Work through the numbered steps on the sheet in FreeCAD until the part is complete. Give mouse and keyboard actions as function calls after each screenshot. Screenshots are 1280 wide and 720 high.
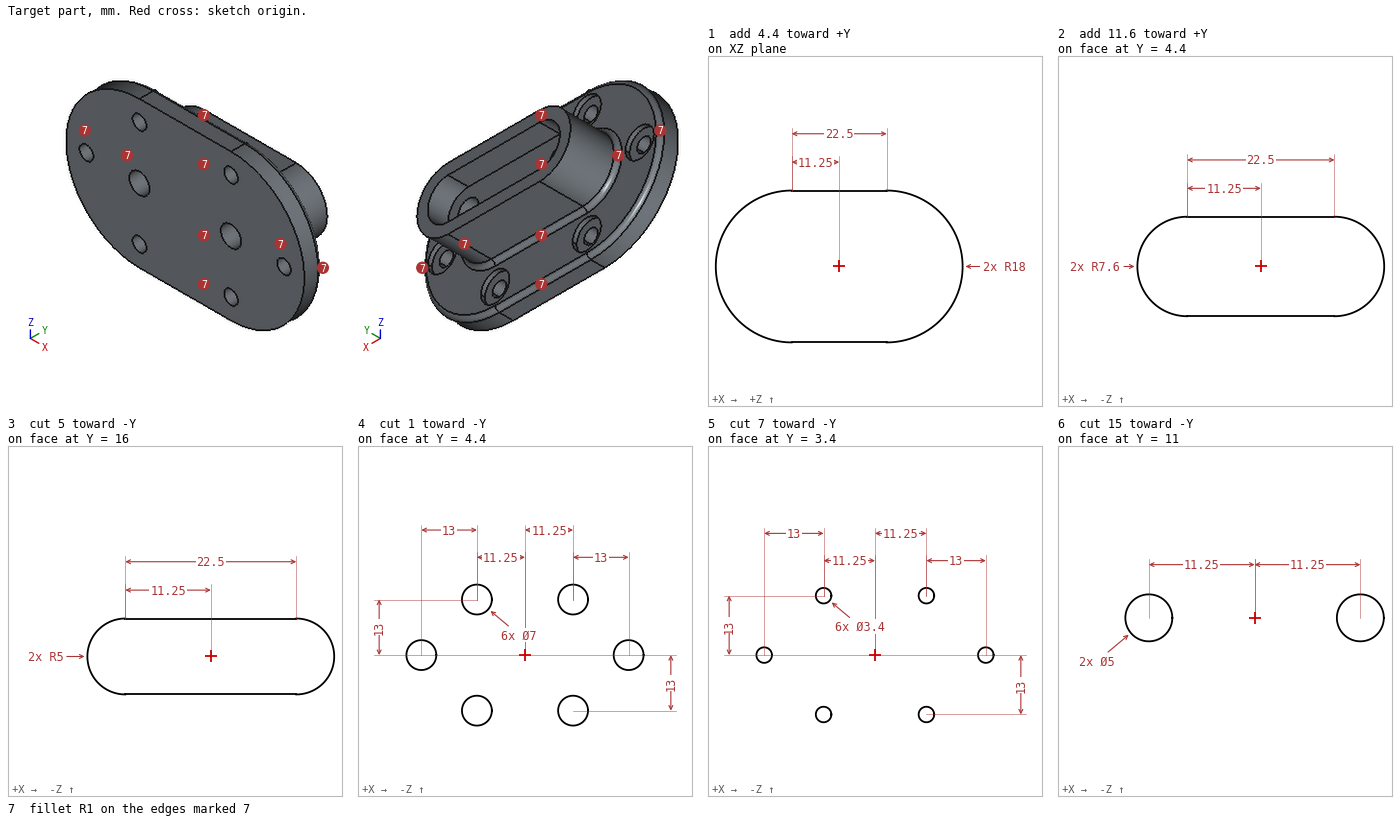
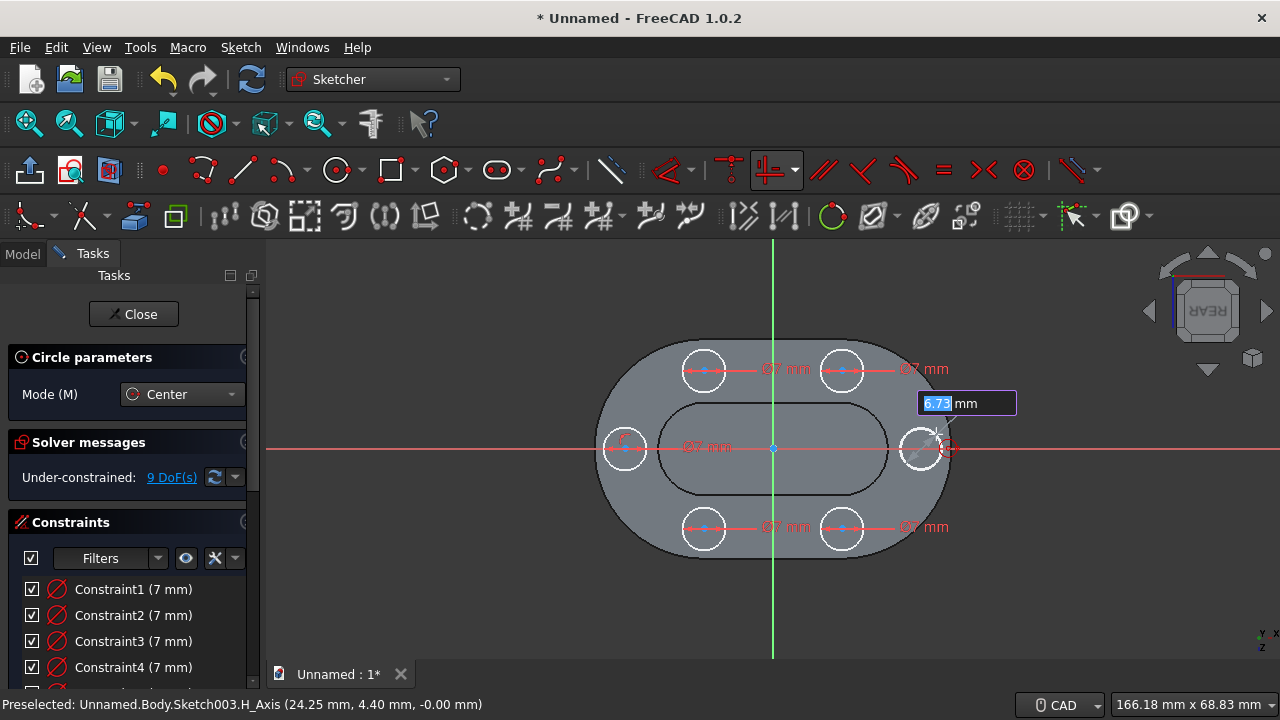
text(7)
key(Return)
key(Escape)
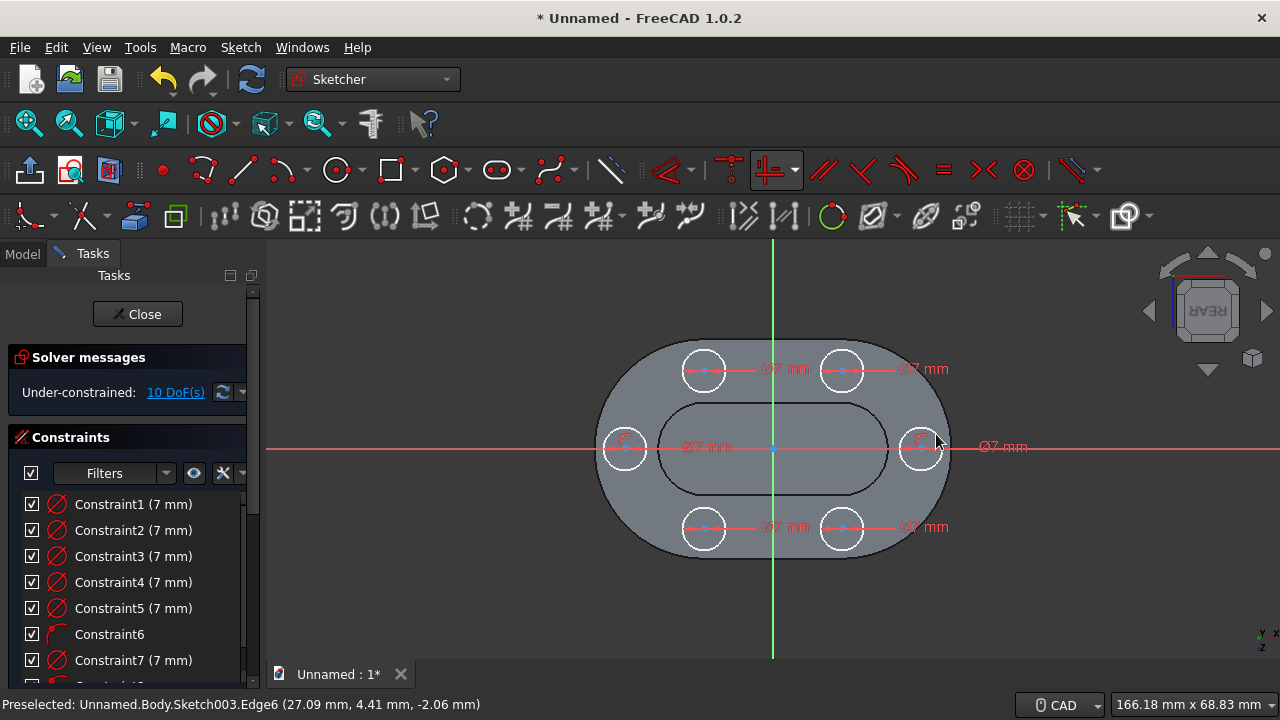
click(704, 371)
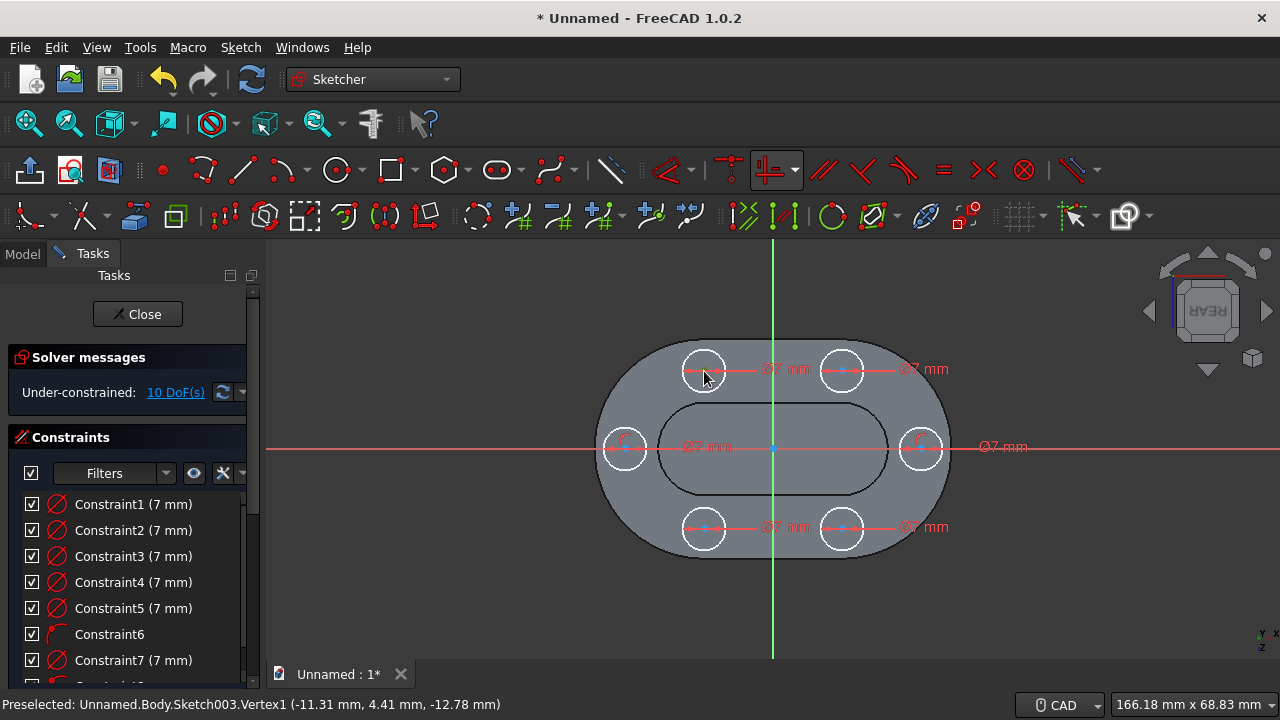
click(842, 371)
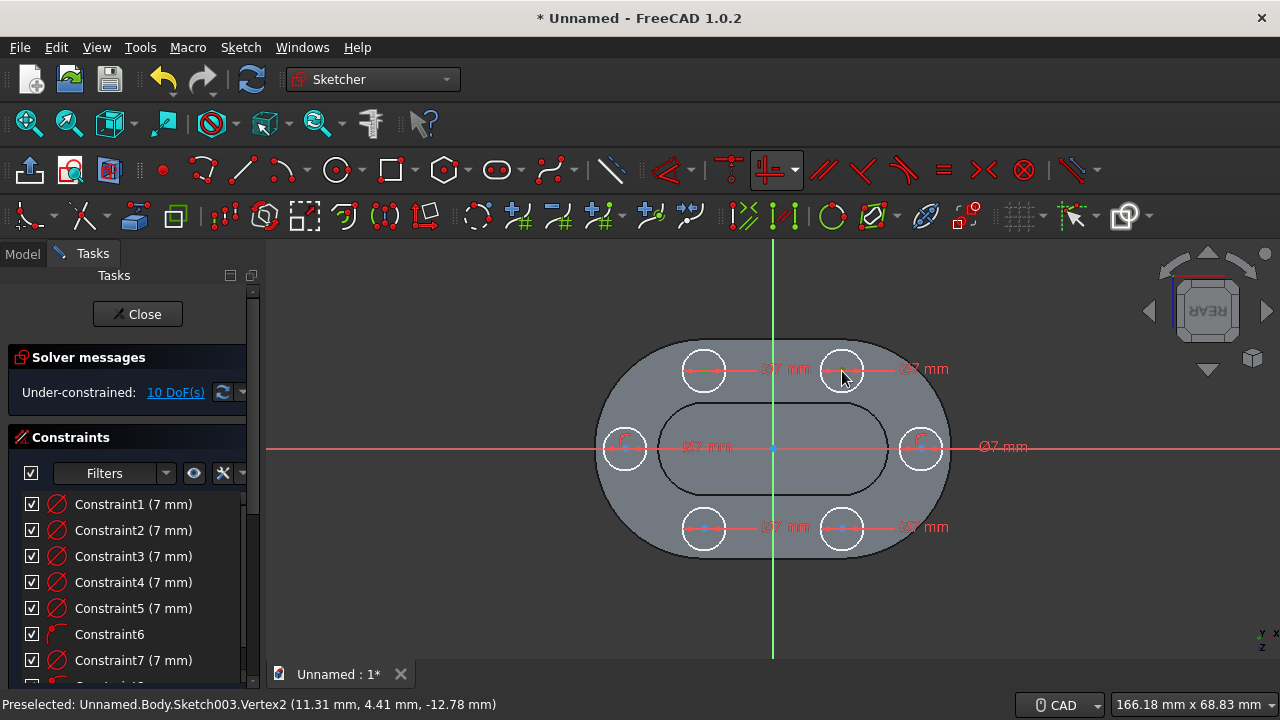
click(798, 170)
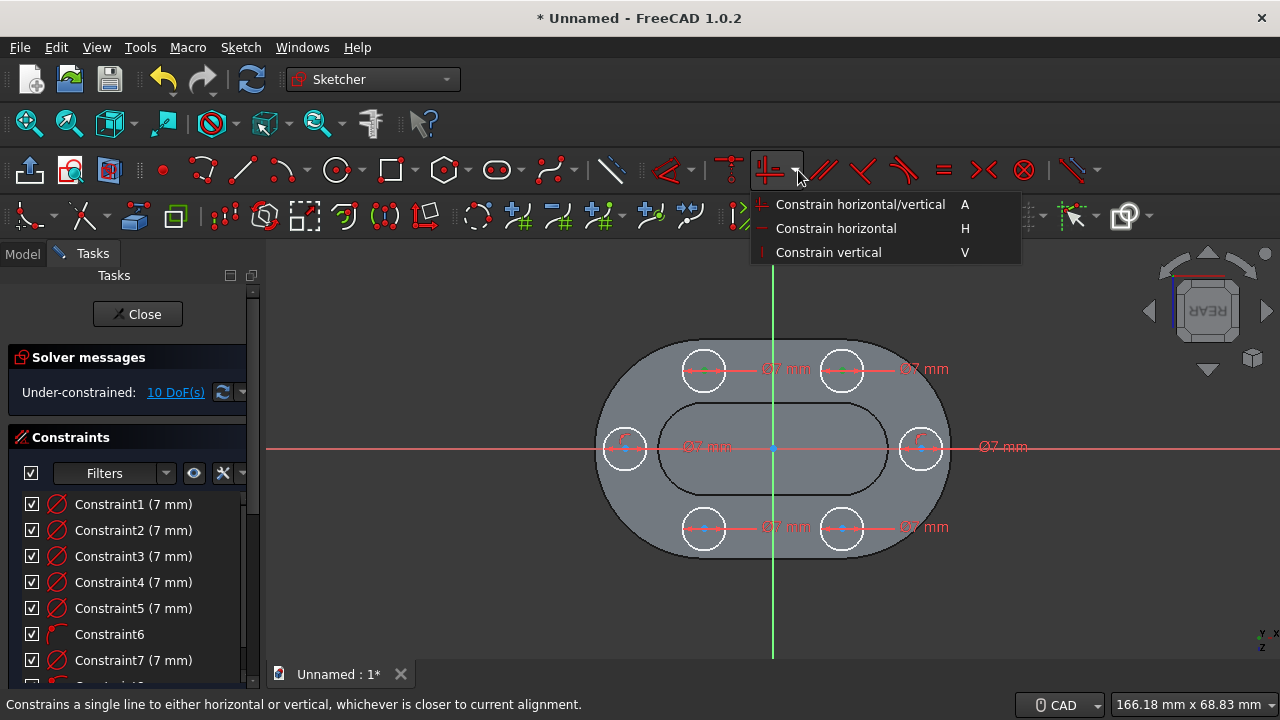
click(886, 228)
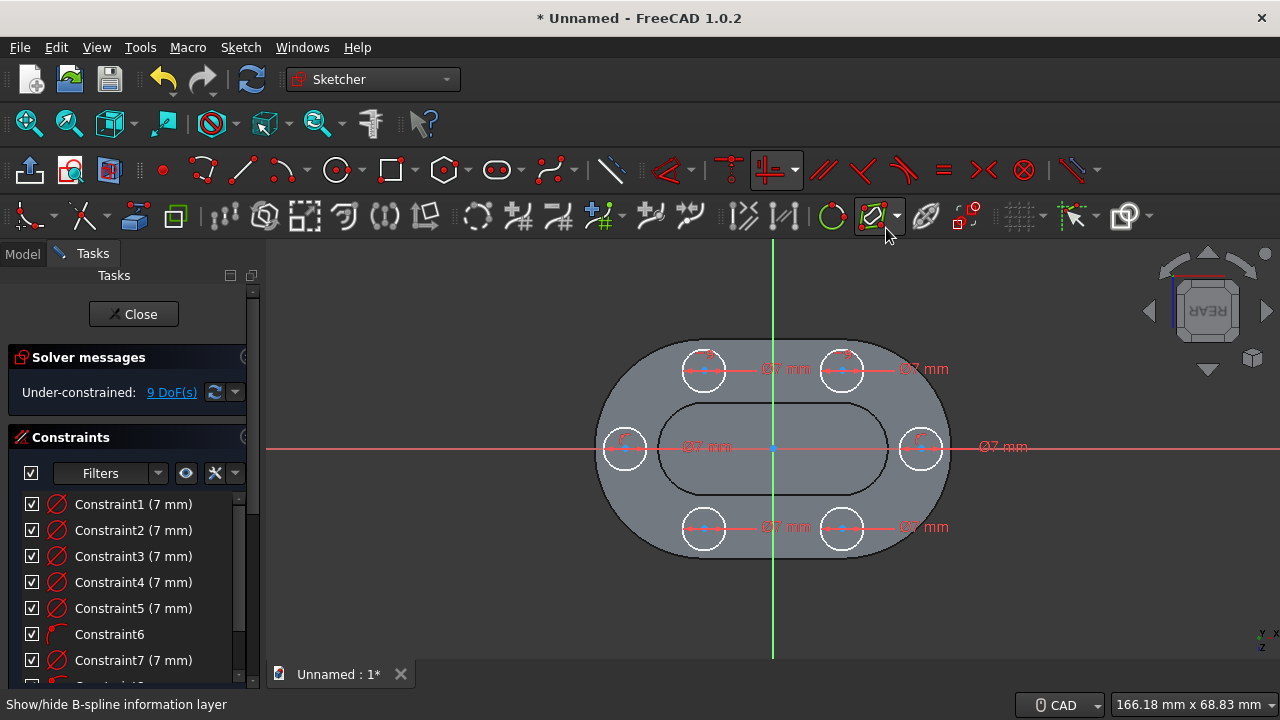
click(842, 371)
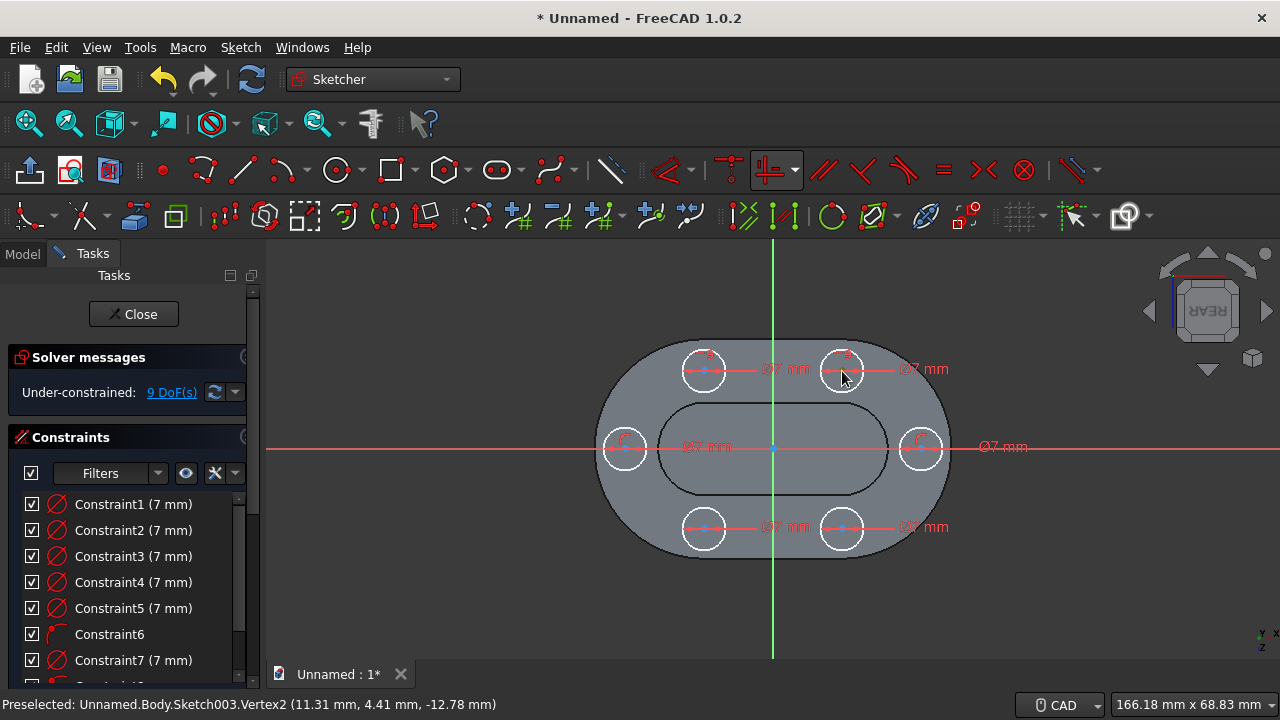
click(842, 529)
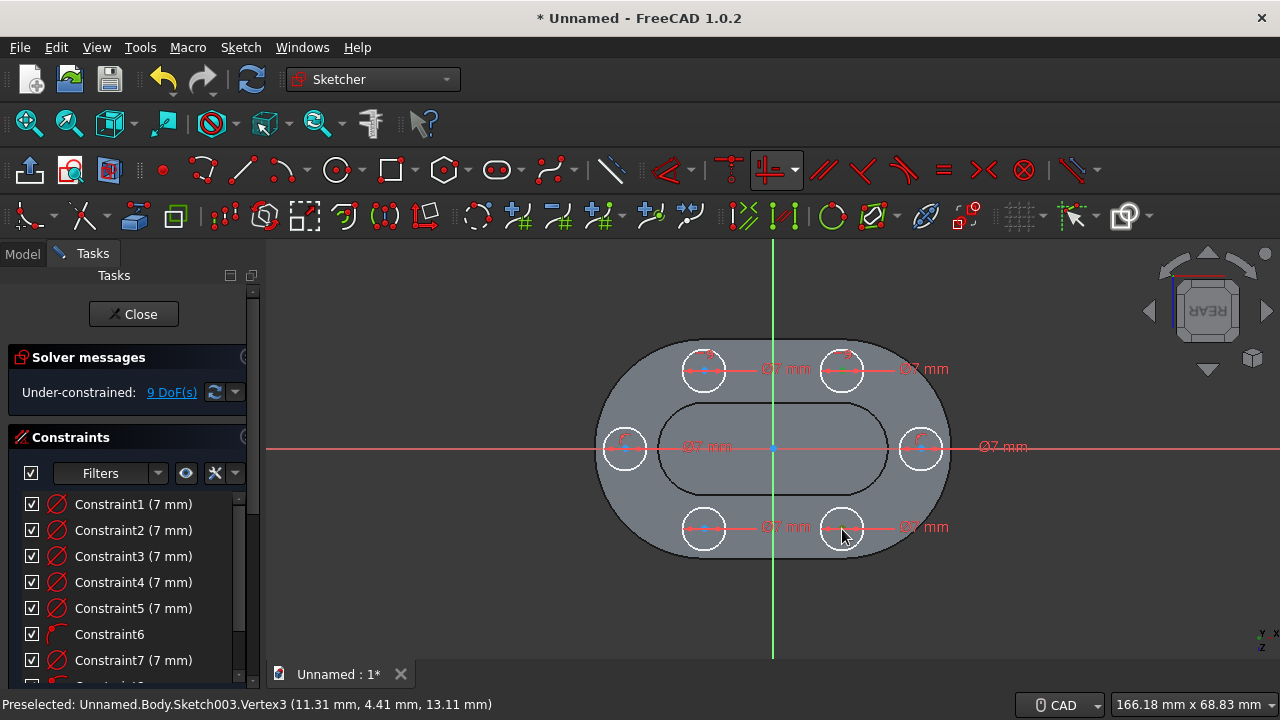
click(798, 170)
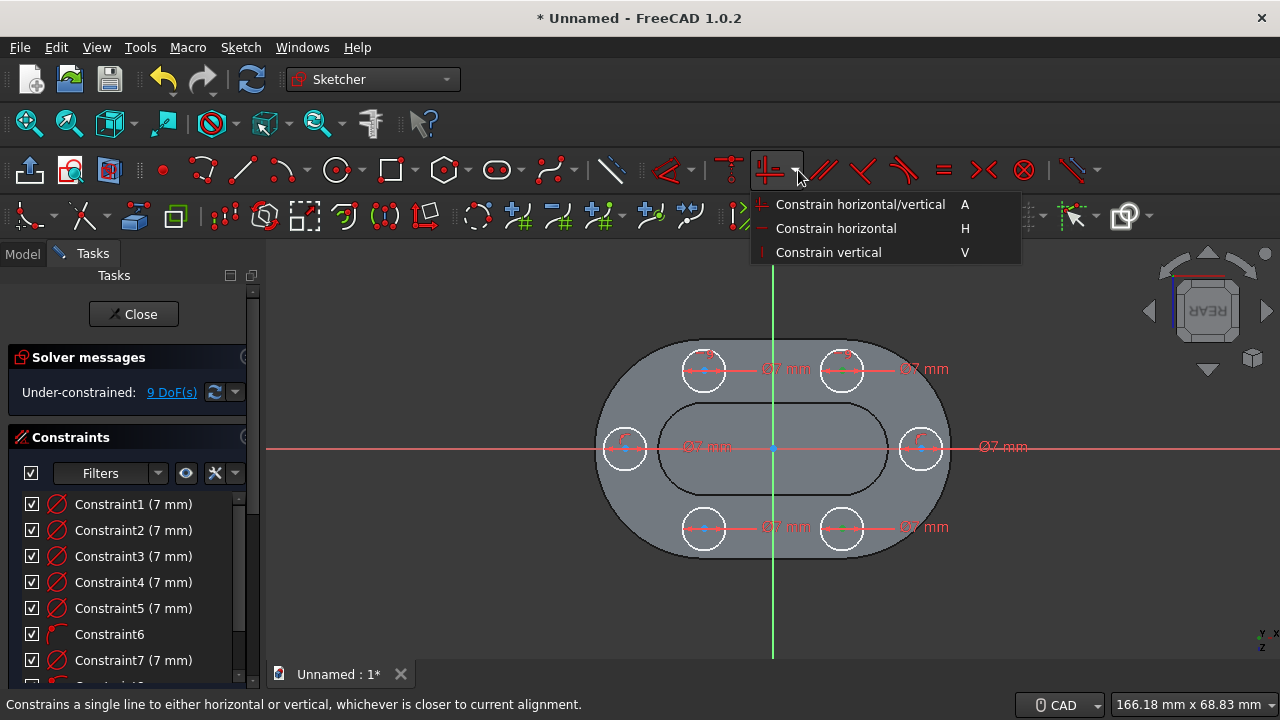
click(886, 252)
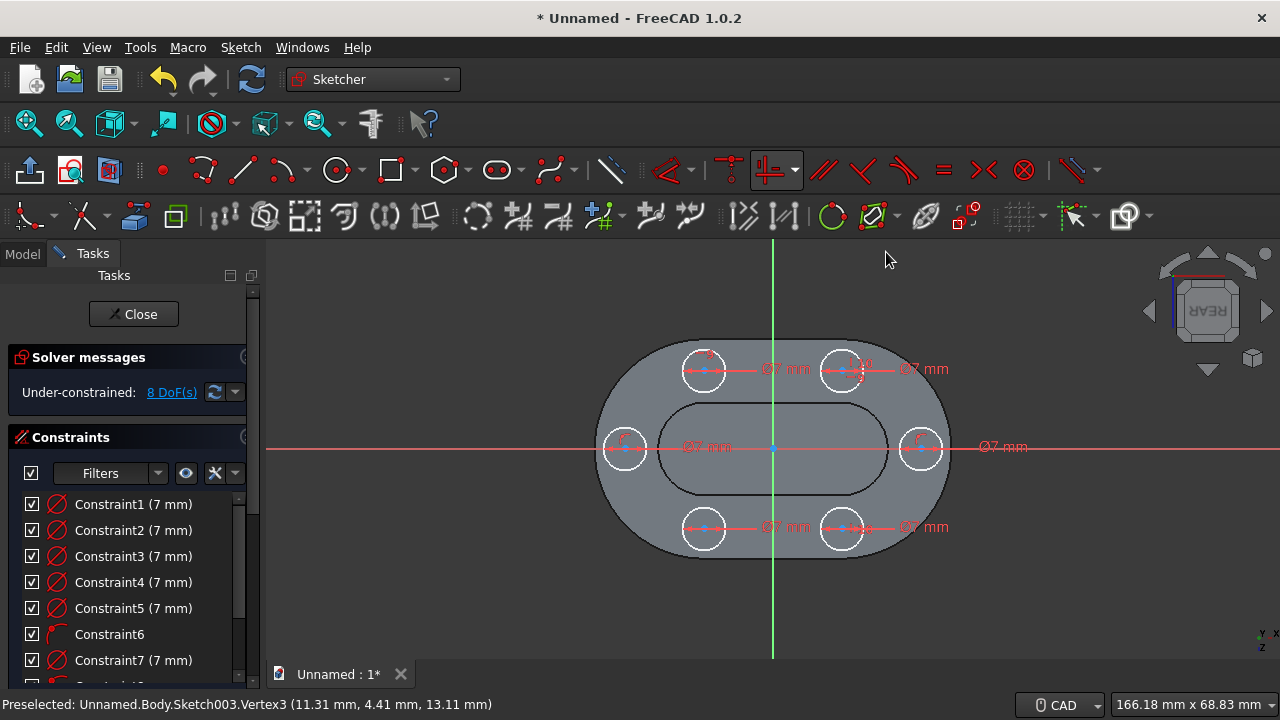
click(704, 371)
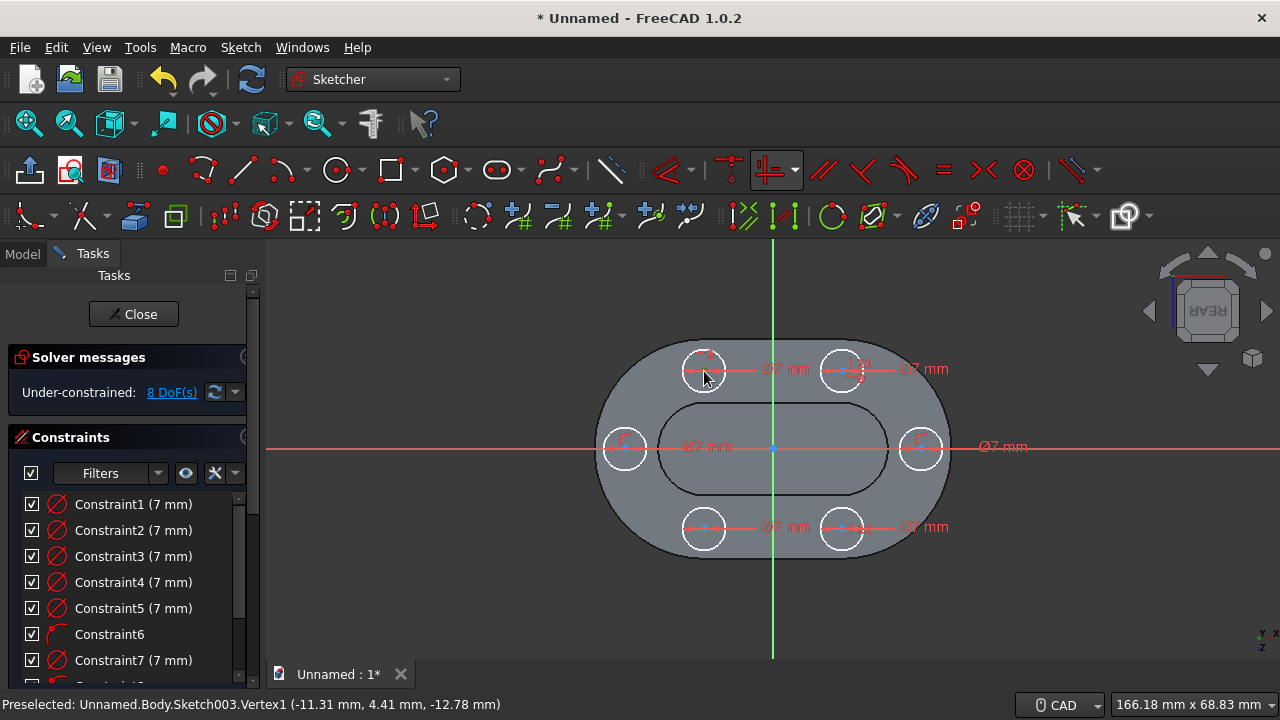
click(704, 529)